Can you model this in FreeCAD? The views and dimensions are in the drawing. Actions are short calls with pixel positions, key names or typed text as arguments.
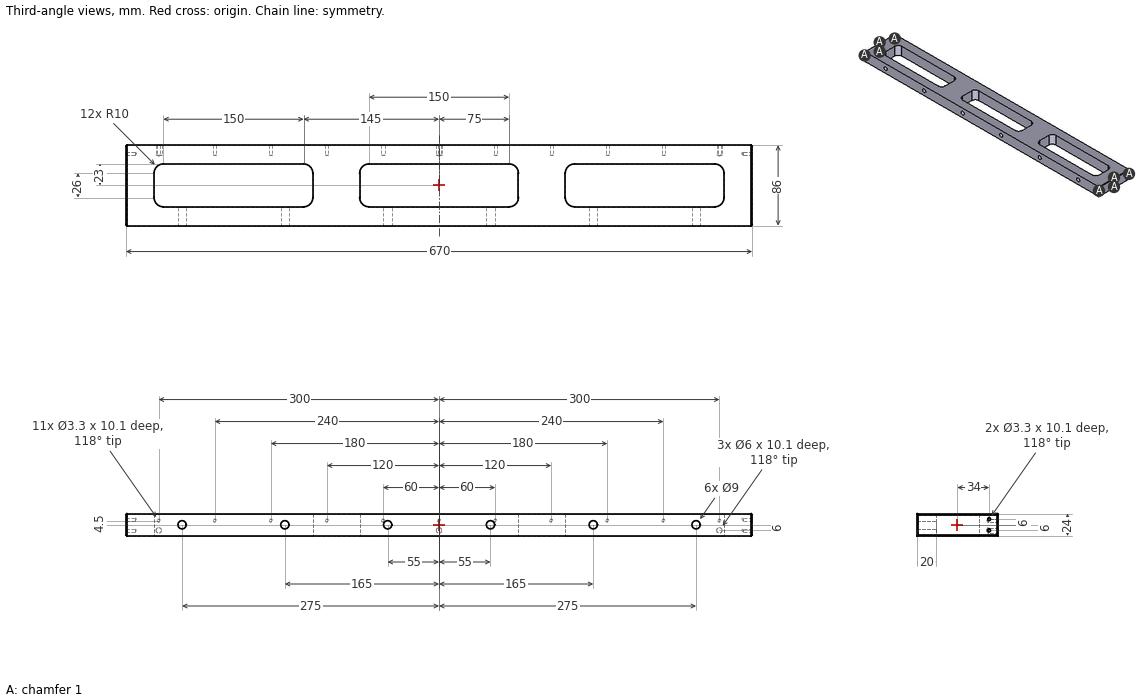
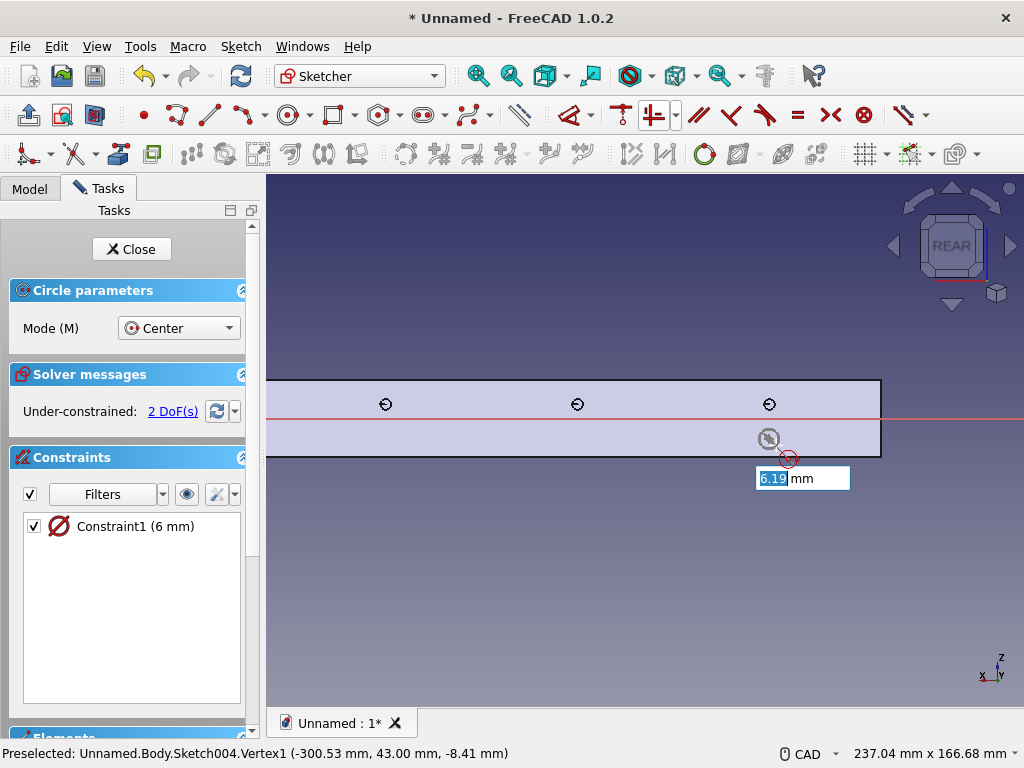
text(6)
key(Return)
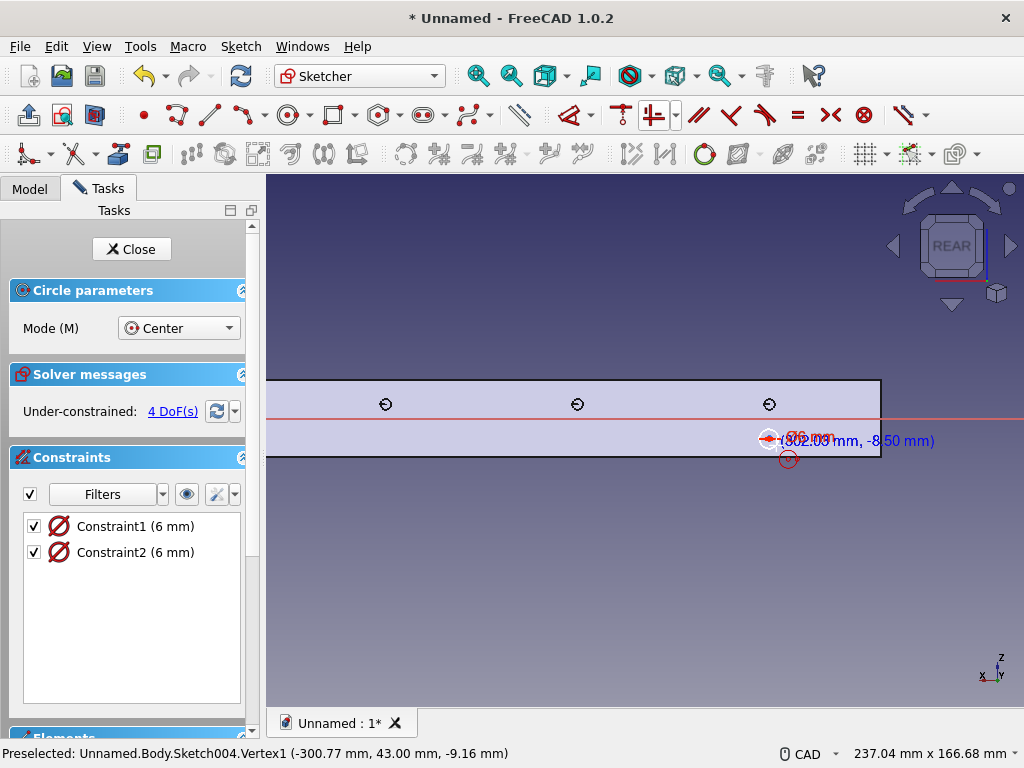
scroll(770, 442, down, 8)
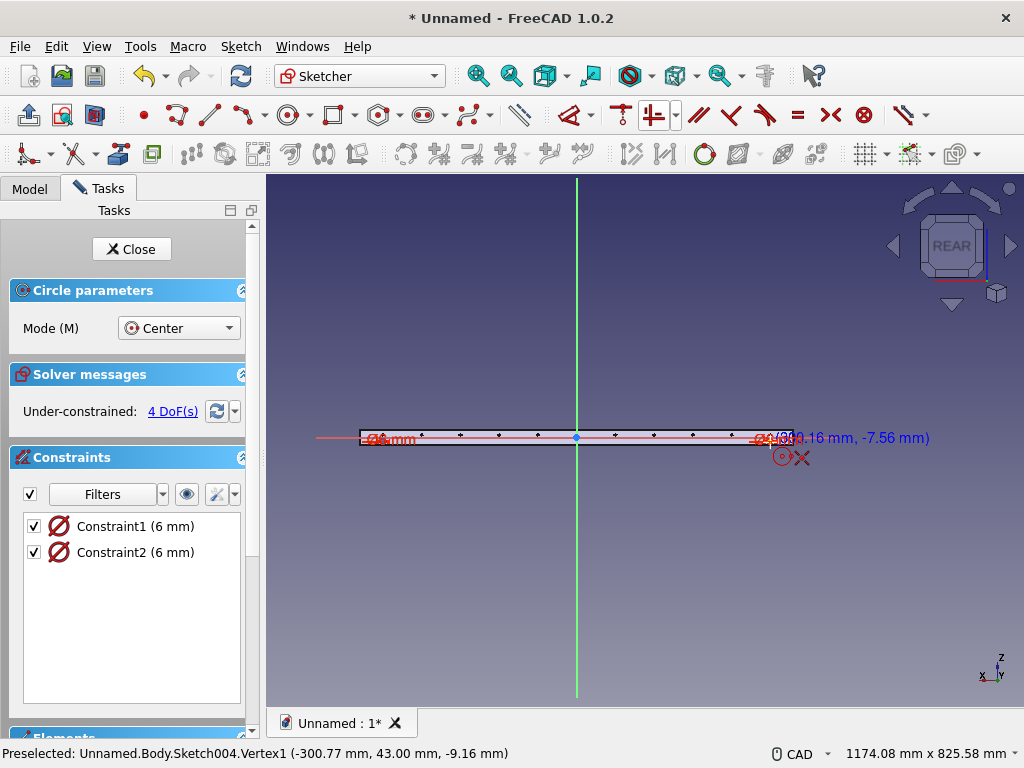
scroll(577, 442, up, 13)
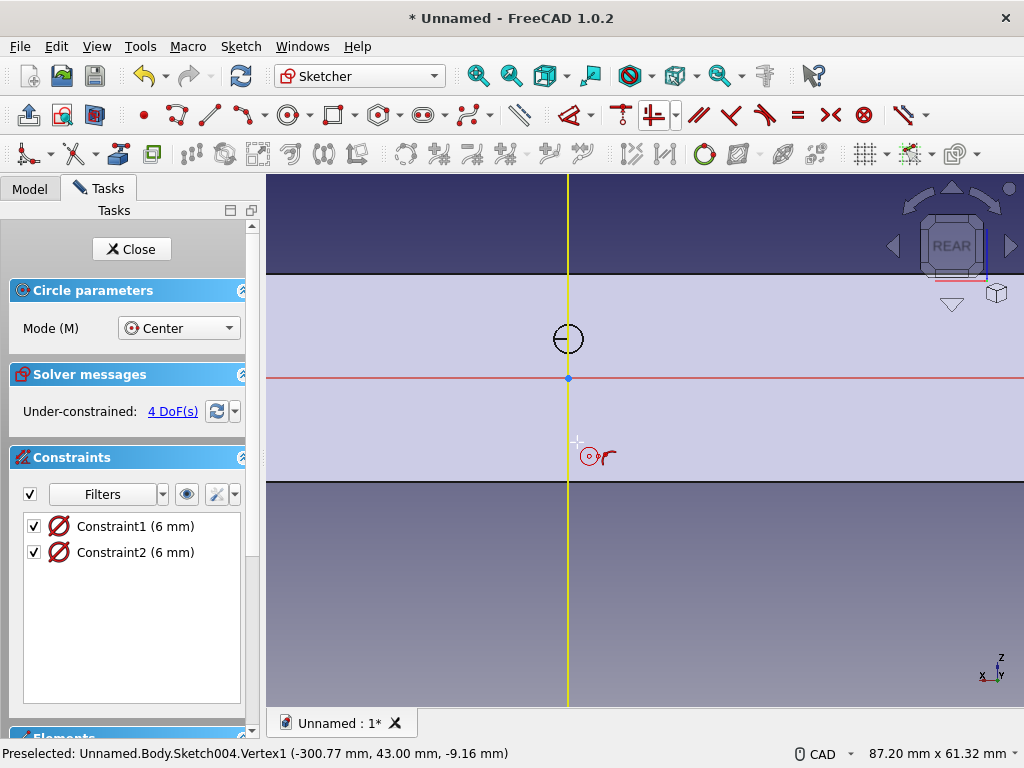
scroll(577, 442, down, 13)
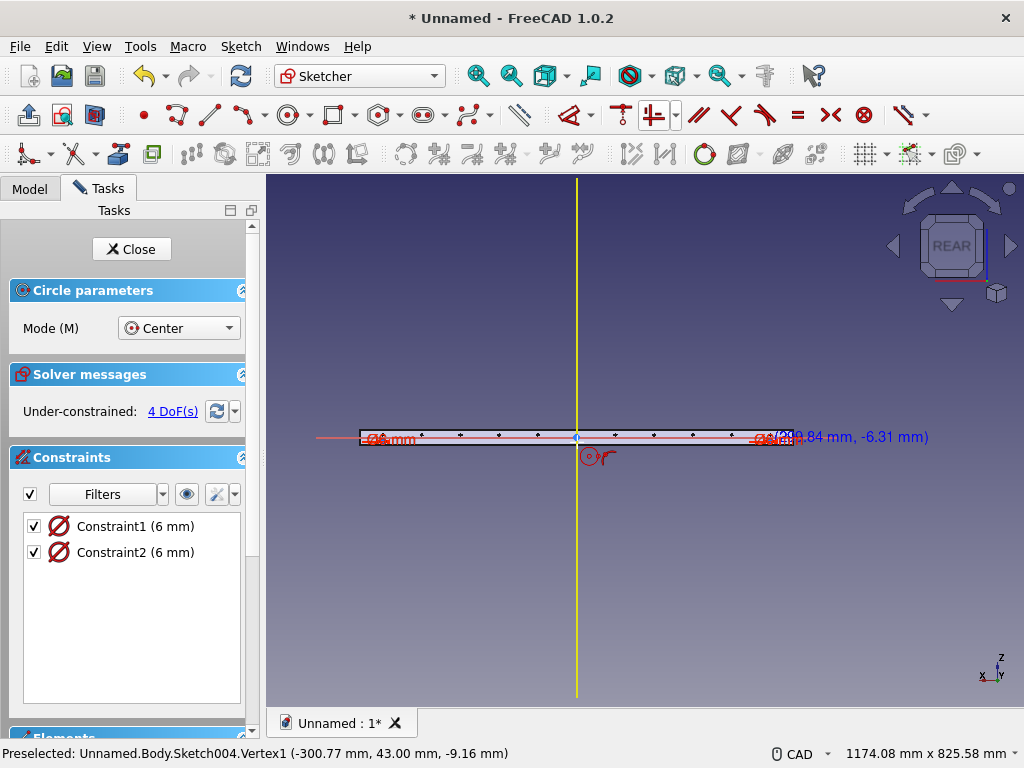
scroll(577, 442, up, 8)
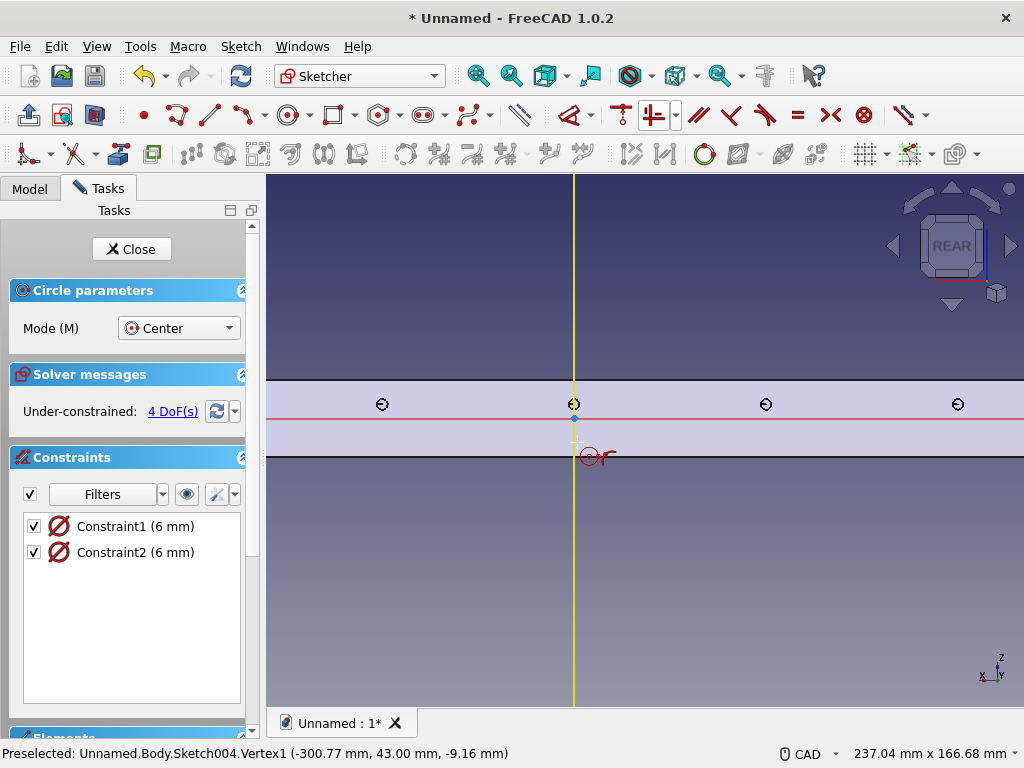
click(574, 438)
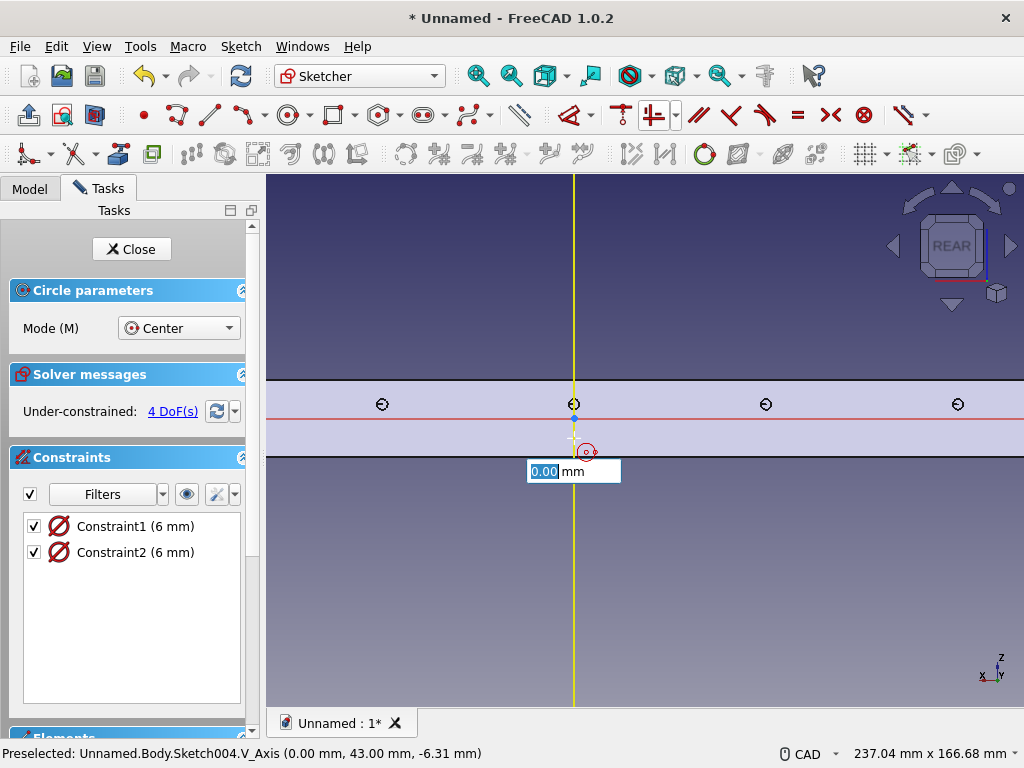
scroll(583, 435, up, 3)
move(583, 434)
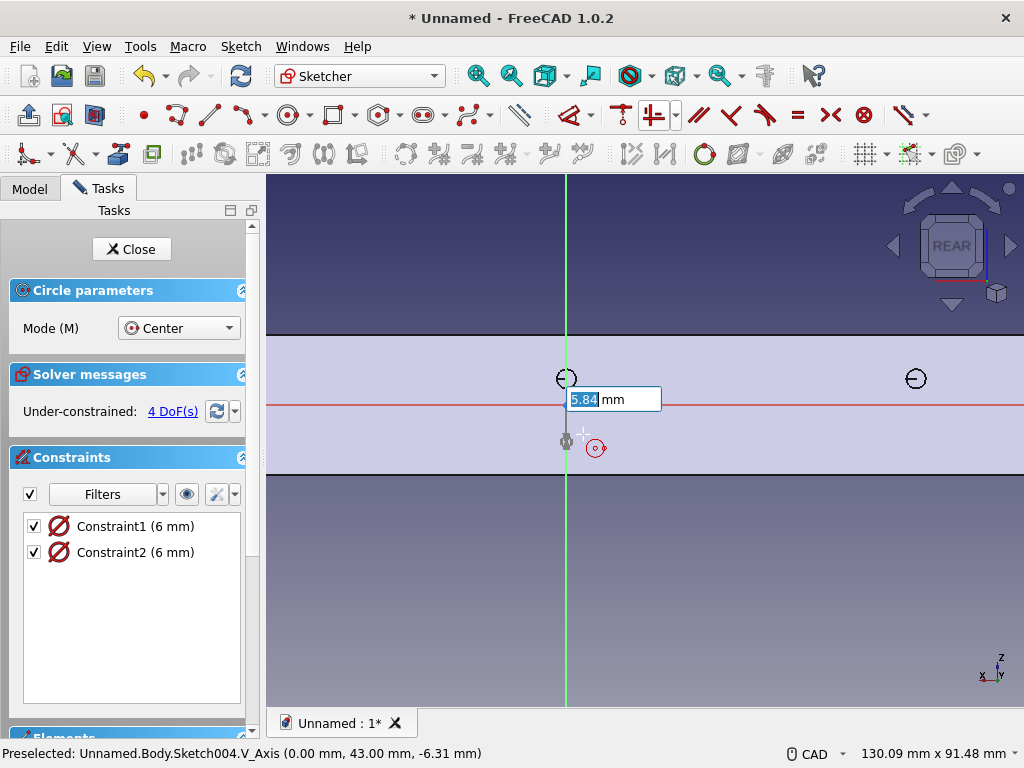
text(6)
key(Return)
key(Escape)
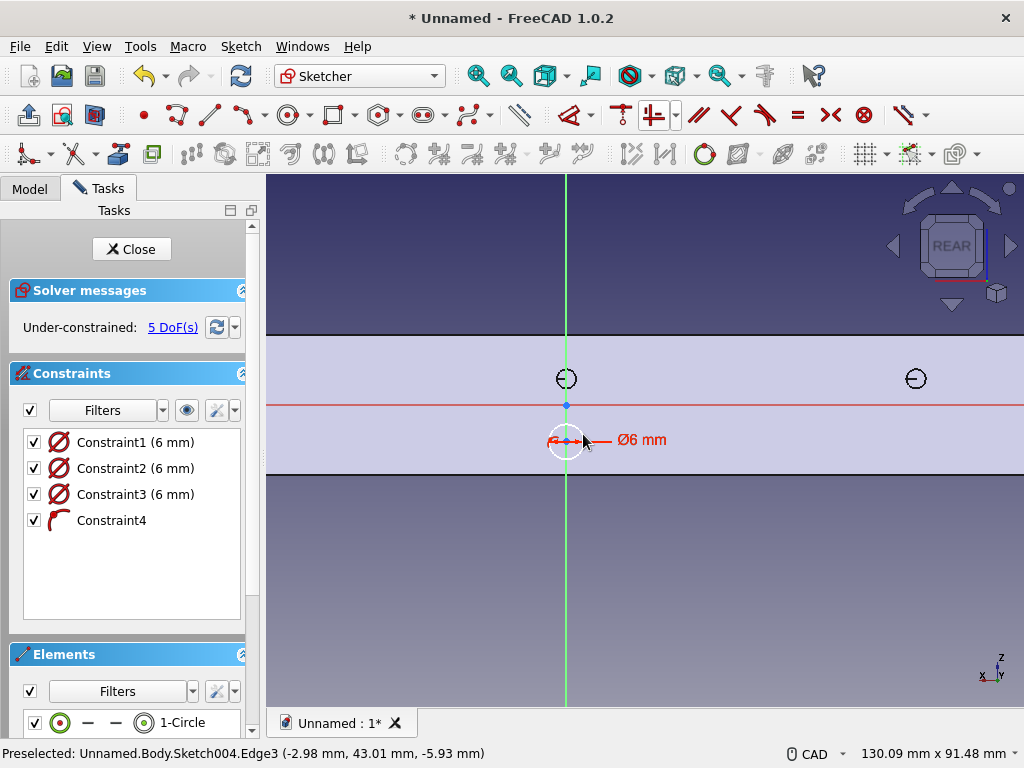
scroll(578, 442, down, 11)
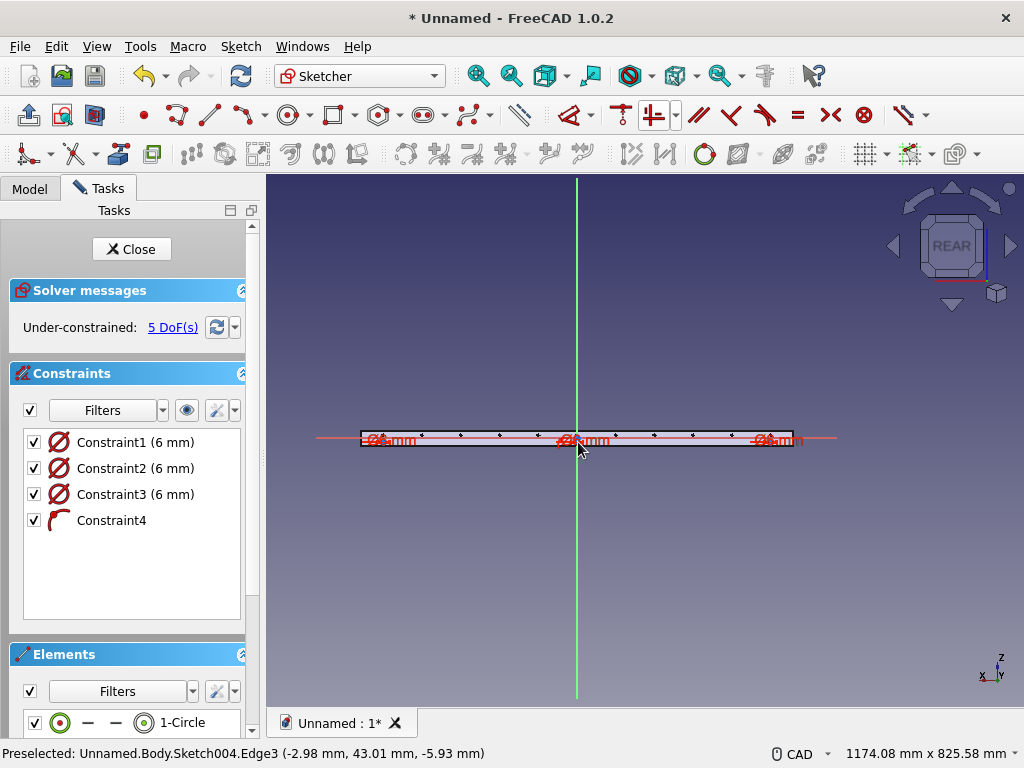
click(383, 442)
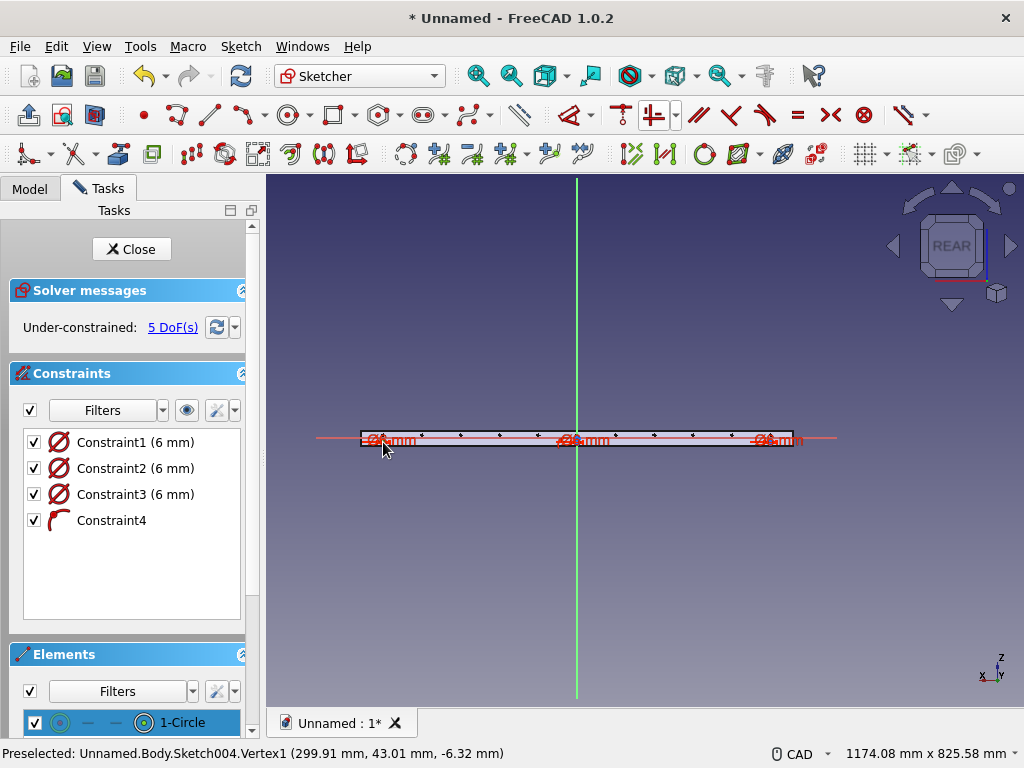
click(771, 442)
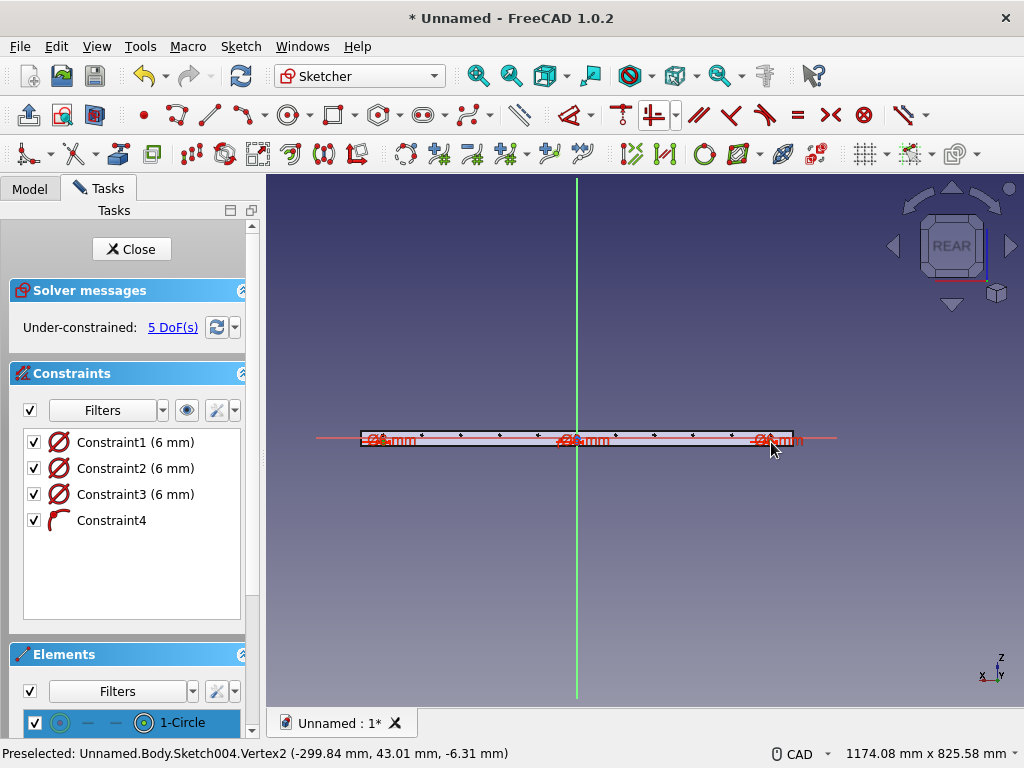
key(h)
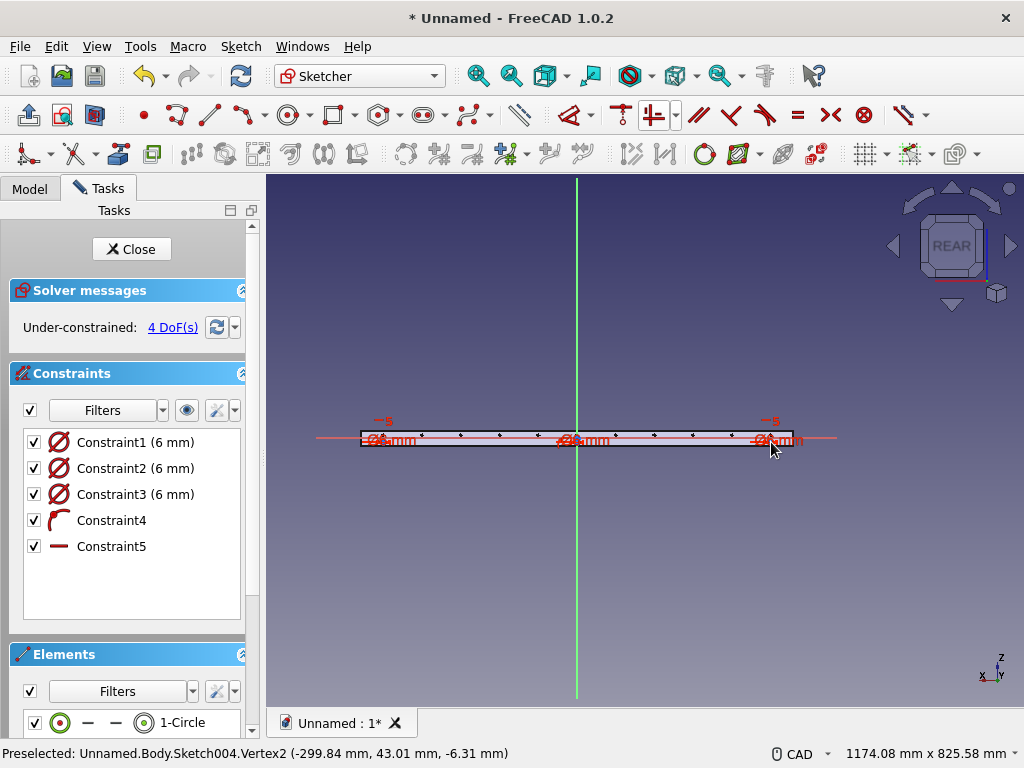
click(383, 442)